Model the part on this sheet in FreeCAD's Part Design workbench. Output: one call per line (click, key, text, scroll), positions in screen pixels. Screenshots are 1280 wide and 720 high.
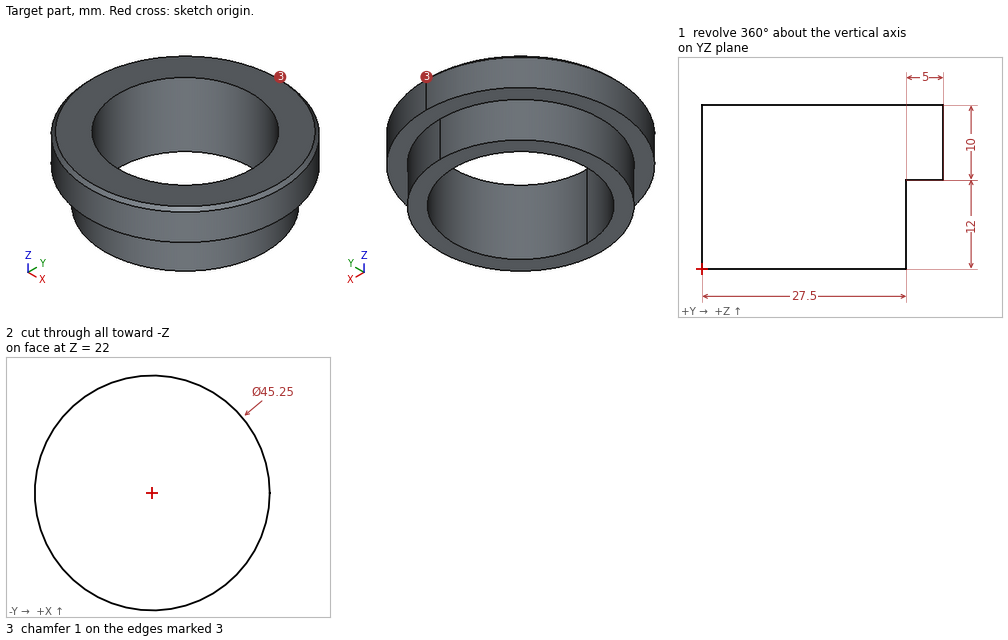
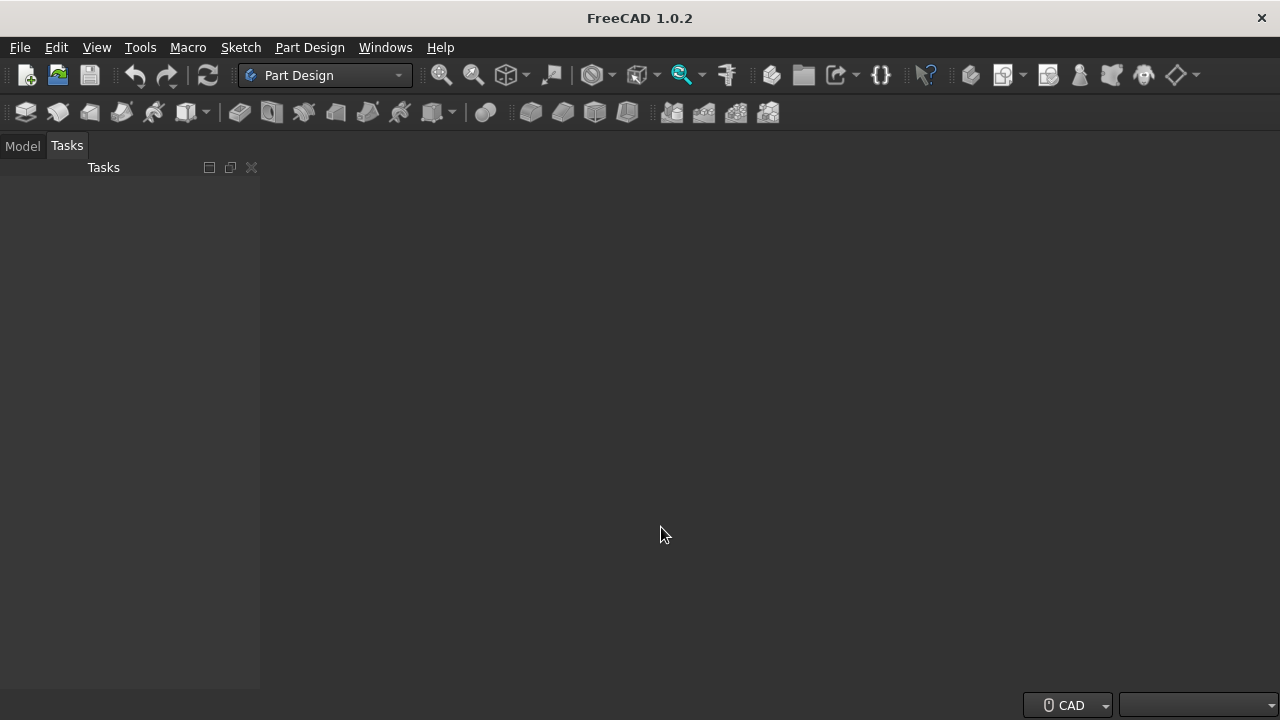
key(ctrl+n)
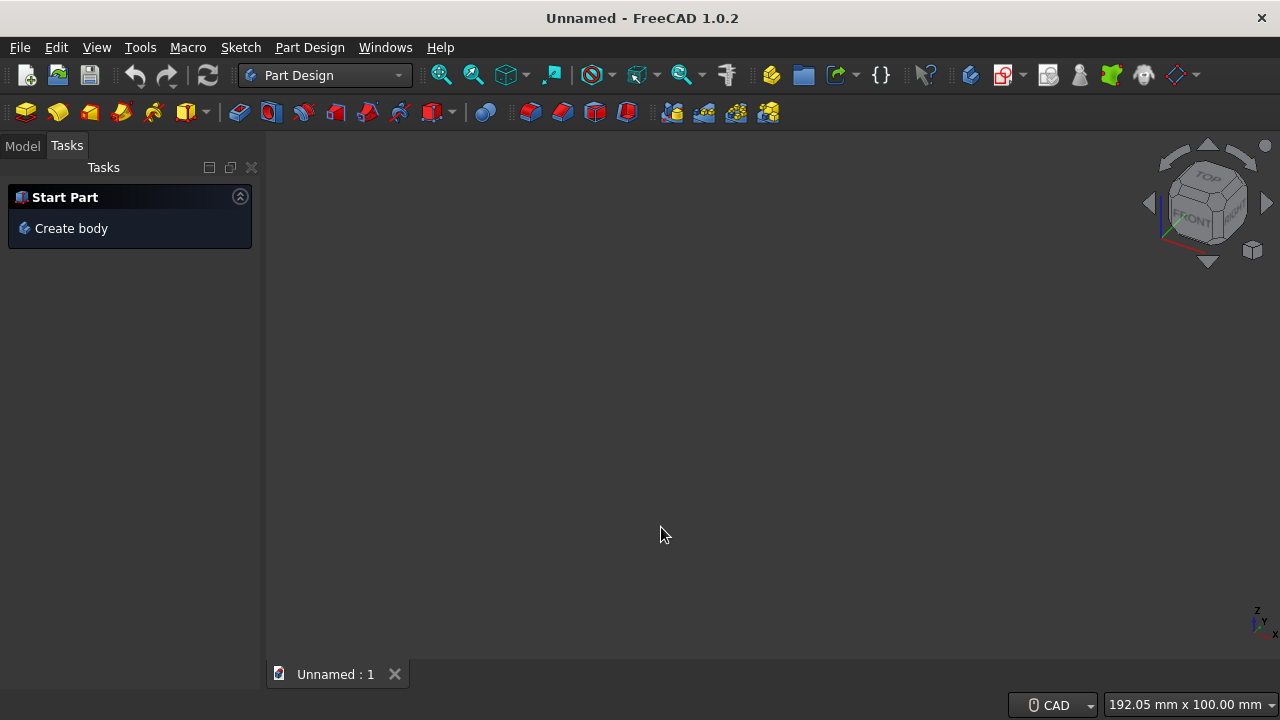
click(1004, 76)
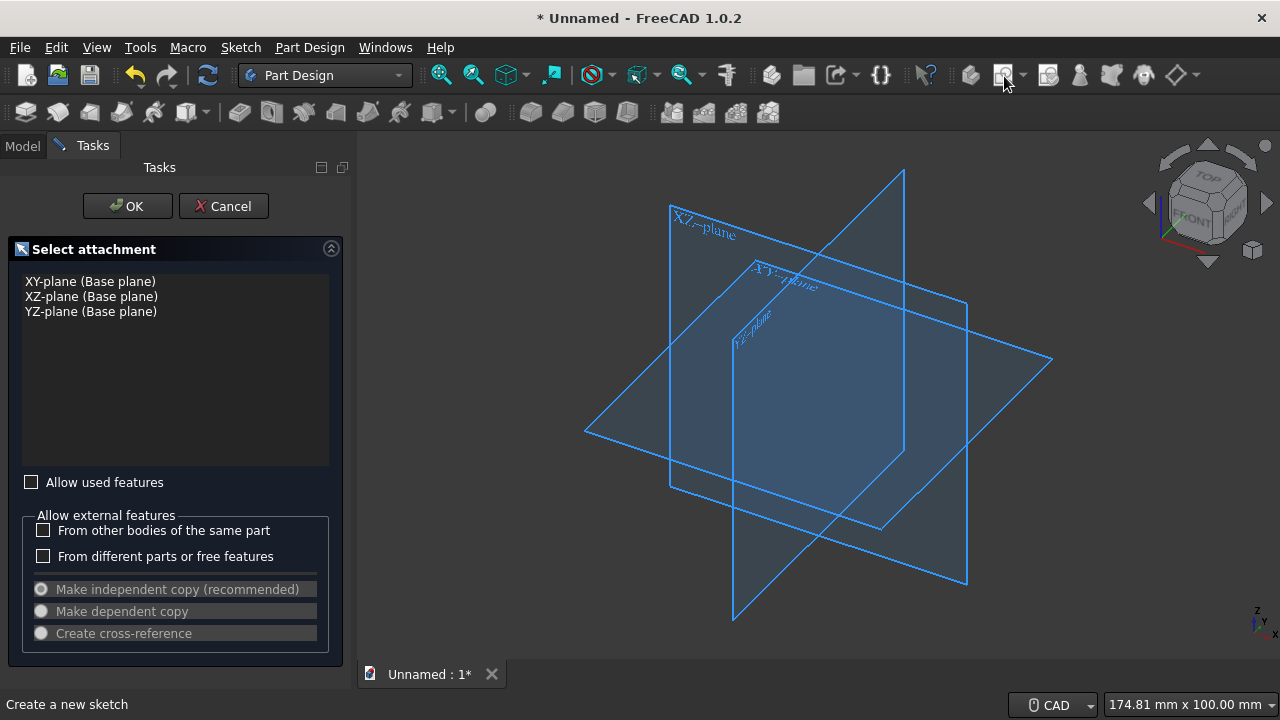
click(82, 312)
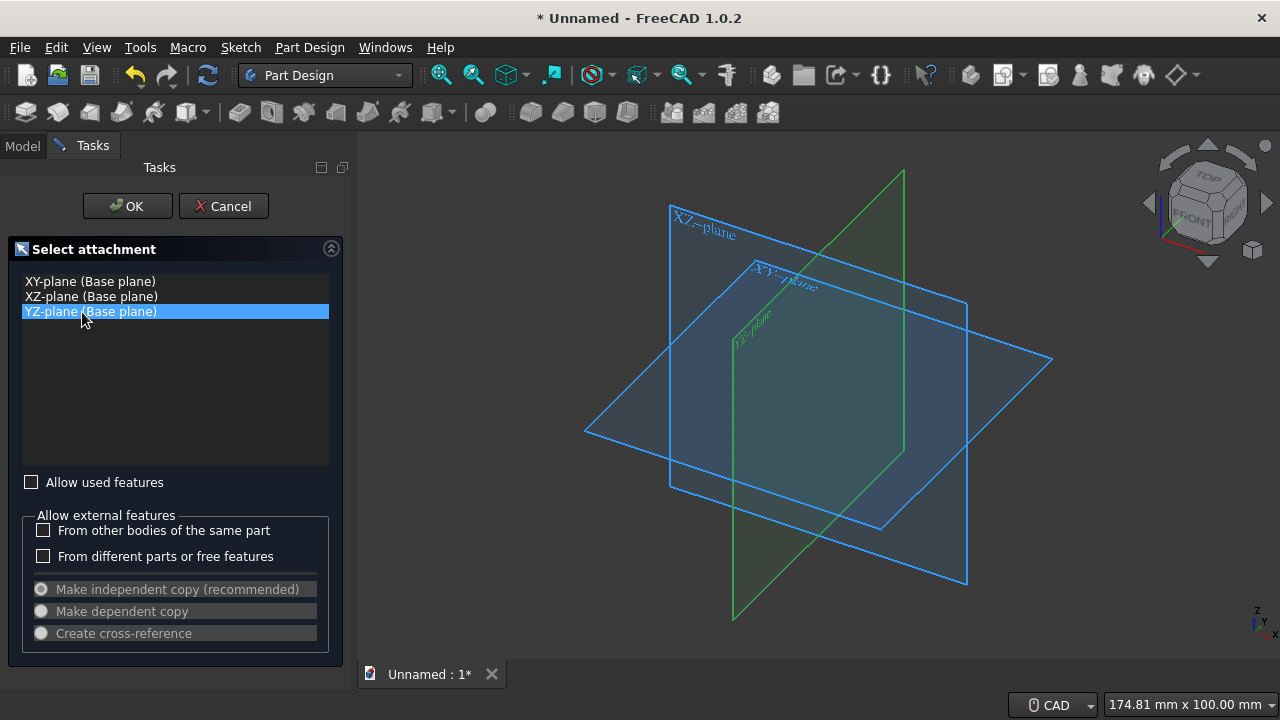
click(128, 206)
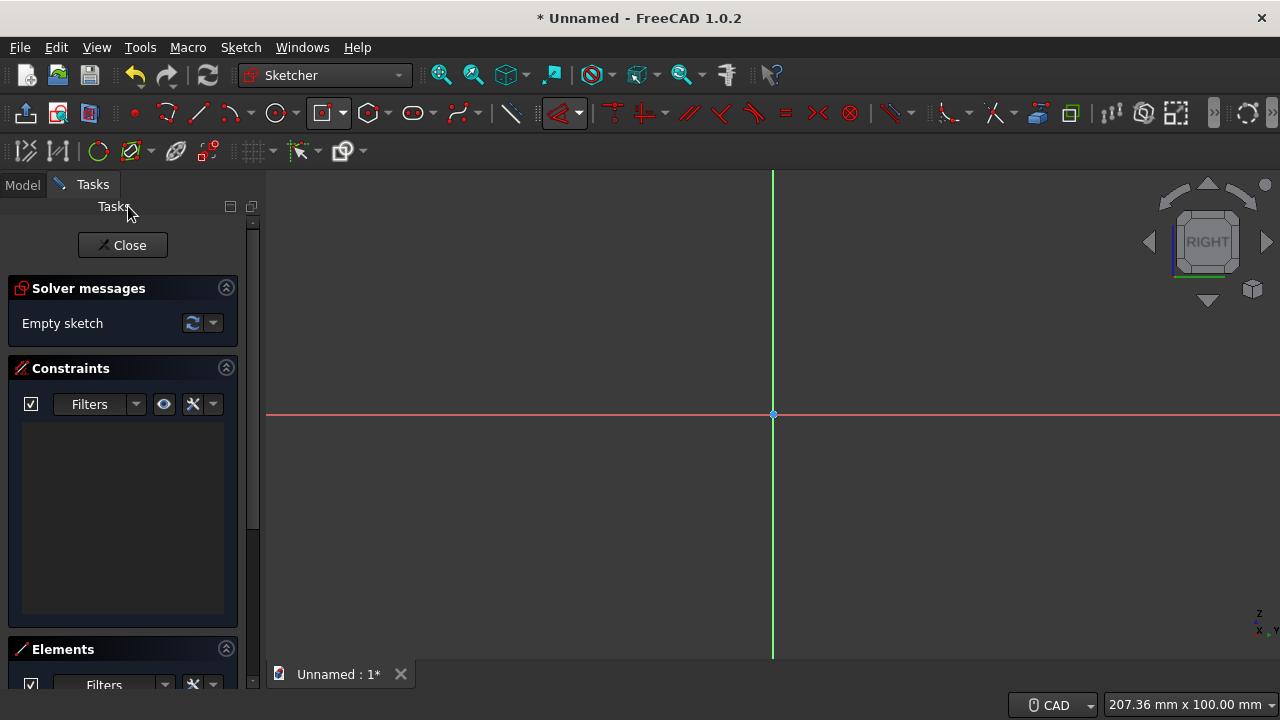
scroll(939, 329, up, 5)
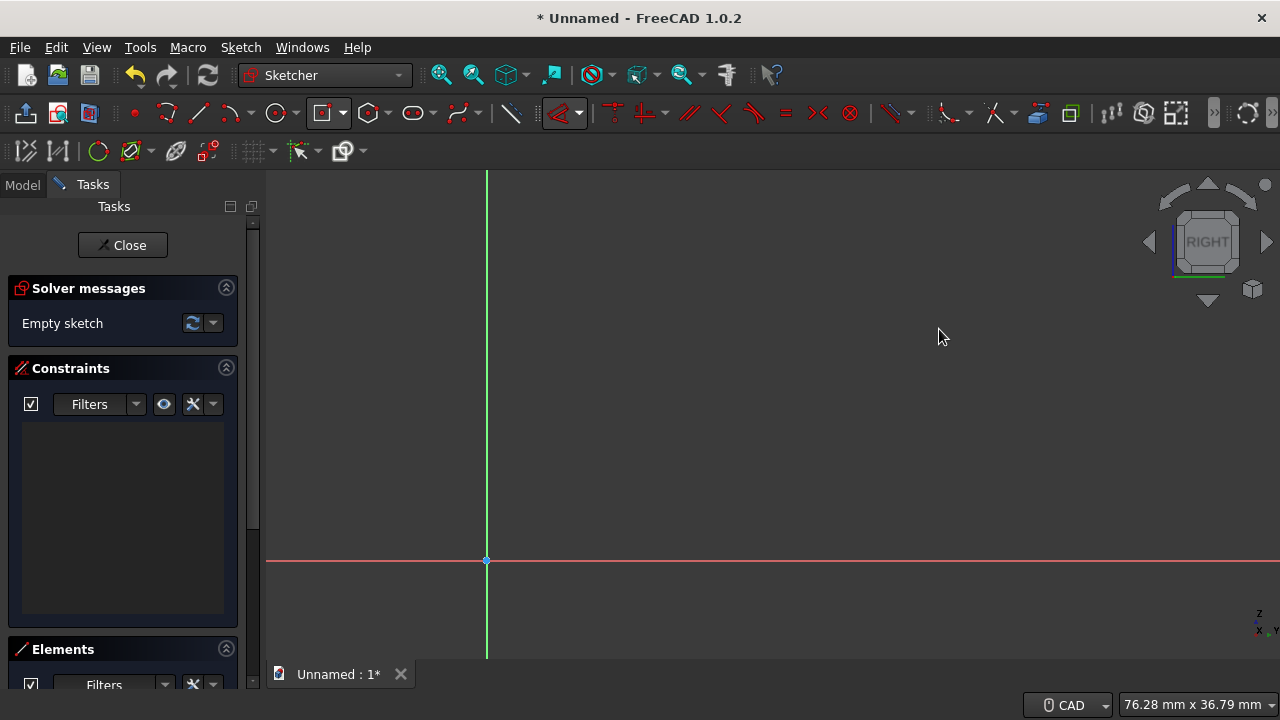
key(g)
key(m)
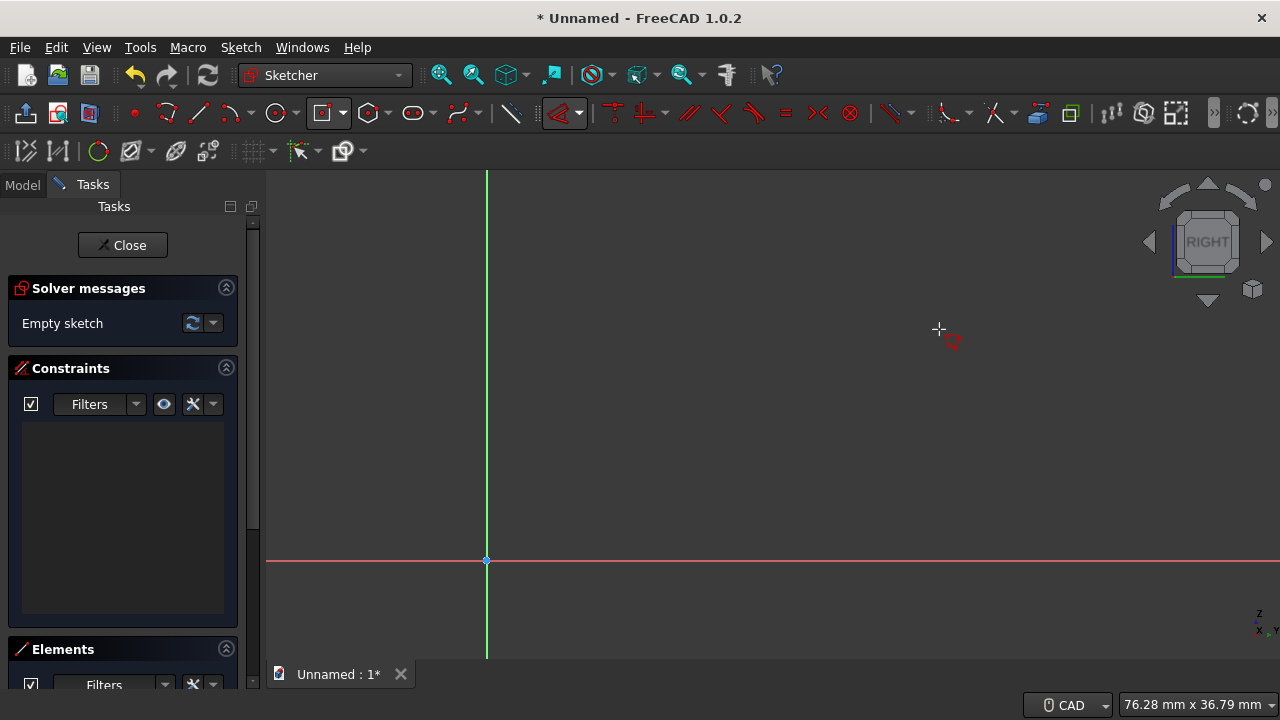
click(487, 561)
click(852, 552)
click(852, 401)
click(919, 401)
click(919, 268)
click(496, 268)
click(487, 561)
key(Escape)
key(Escape)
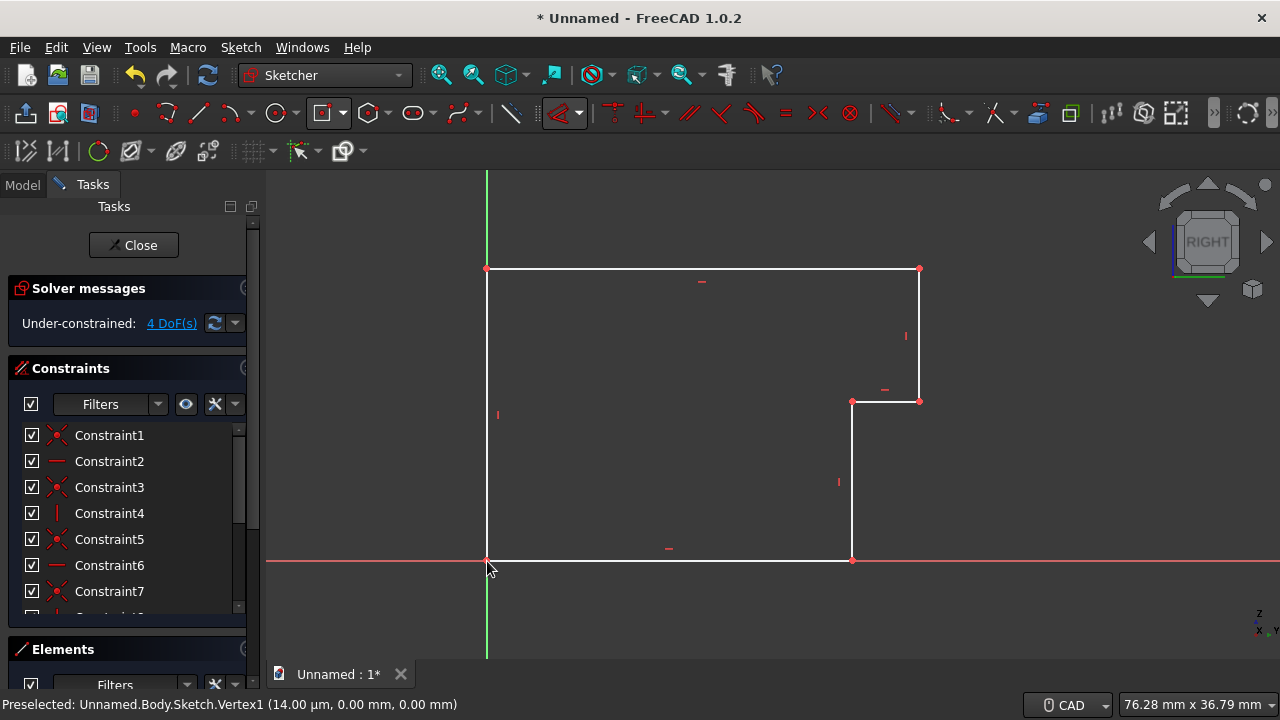
click(872, 402)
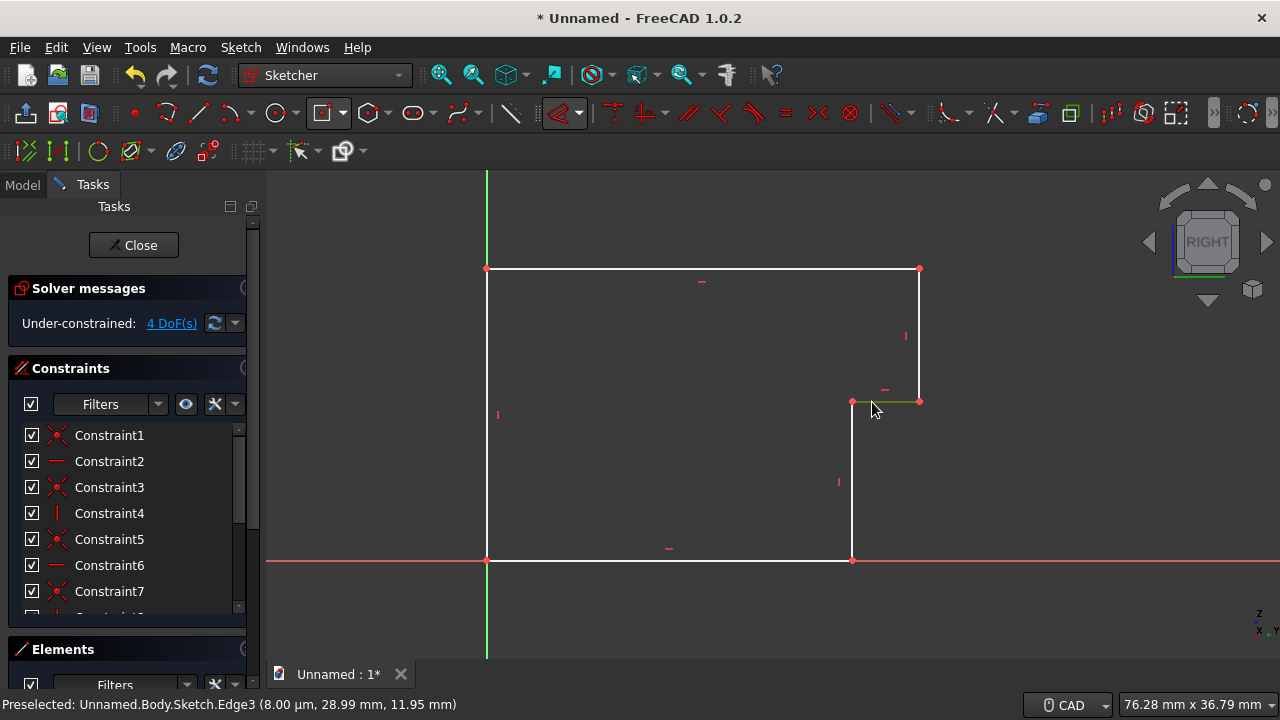
key(l)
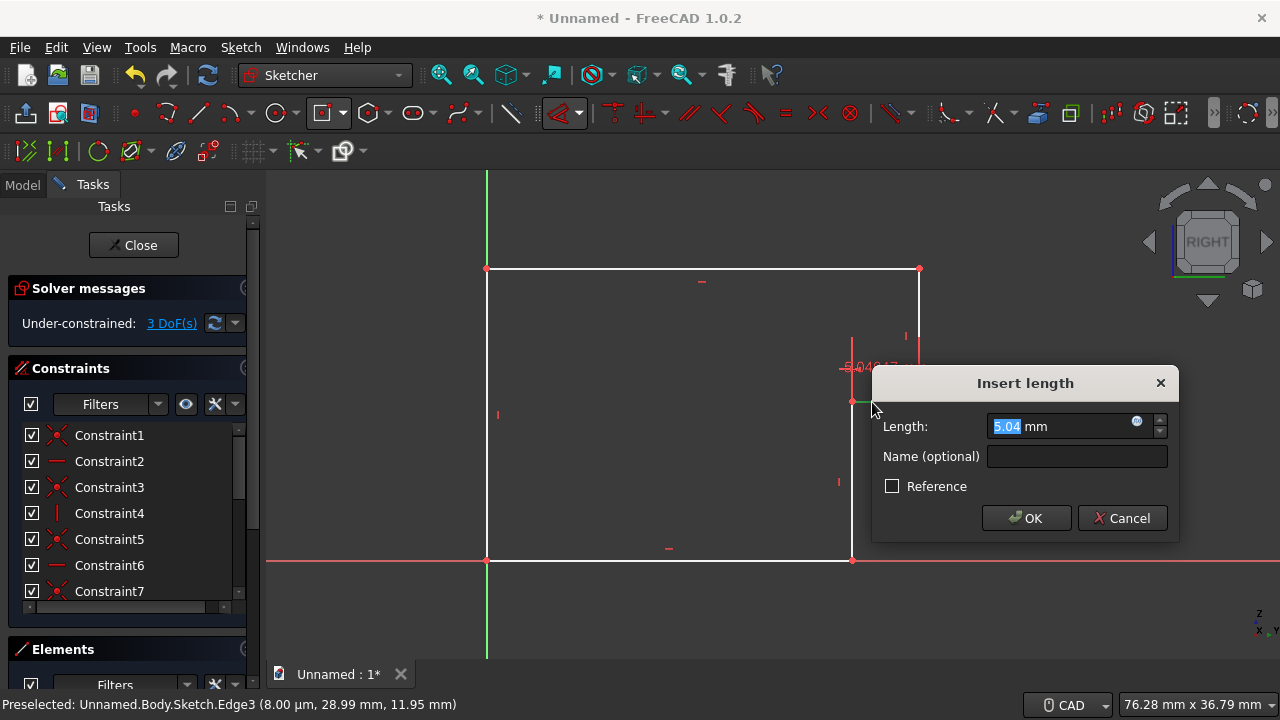
text(5)
key(Return)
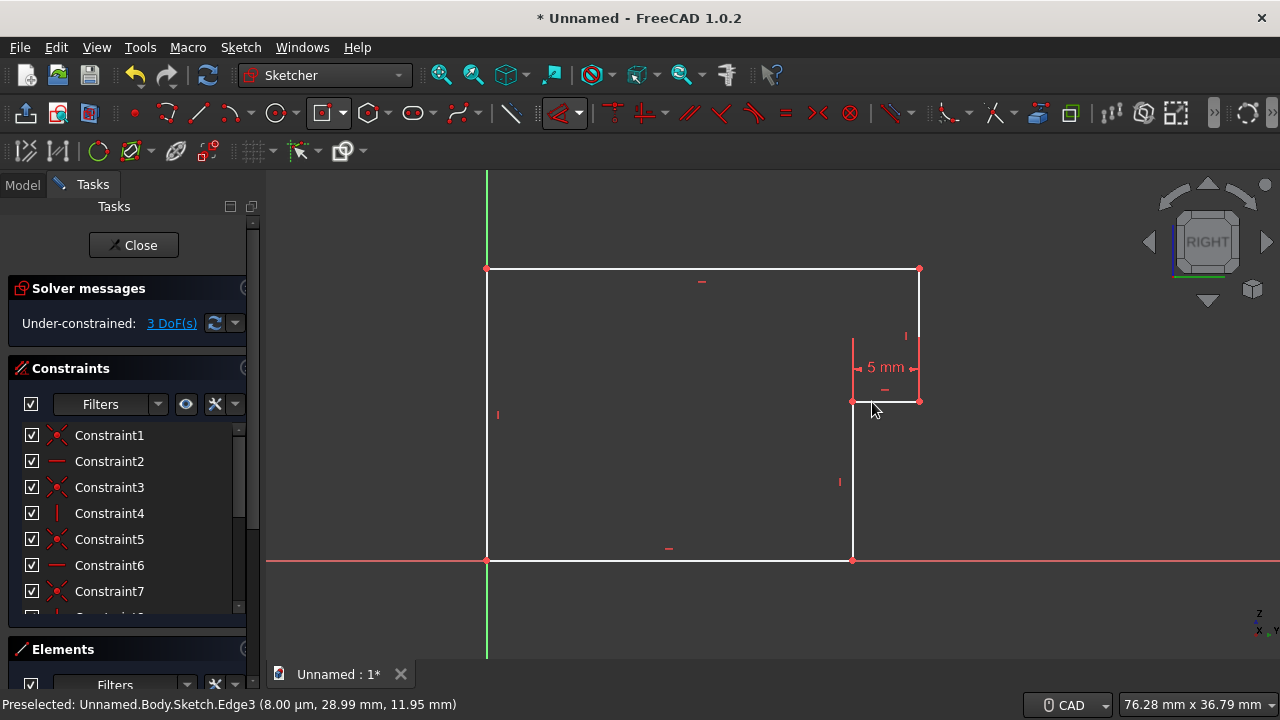
click(853, 513)